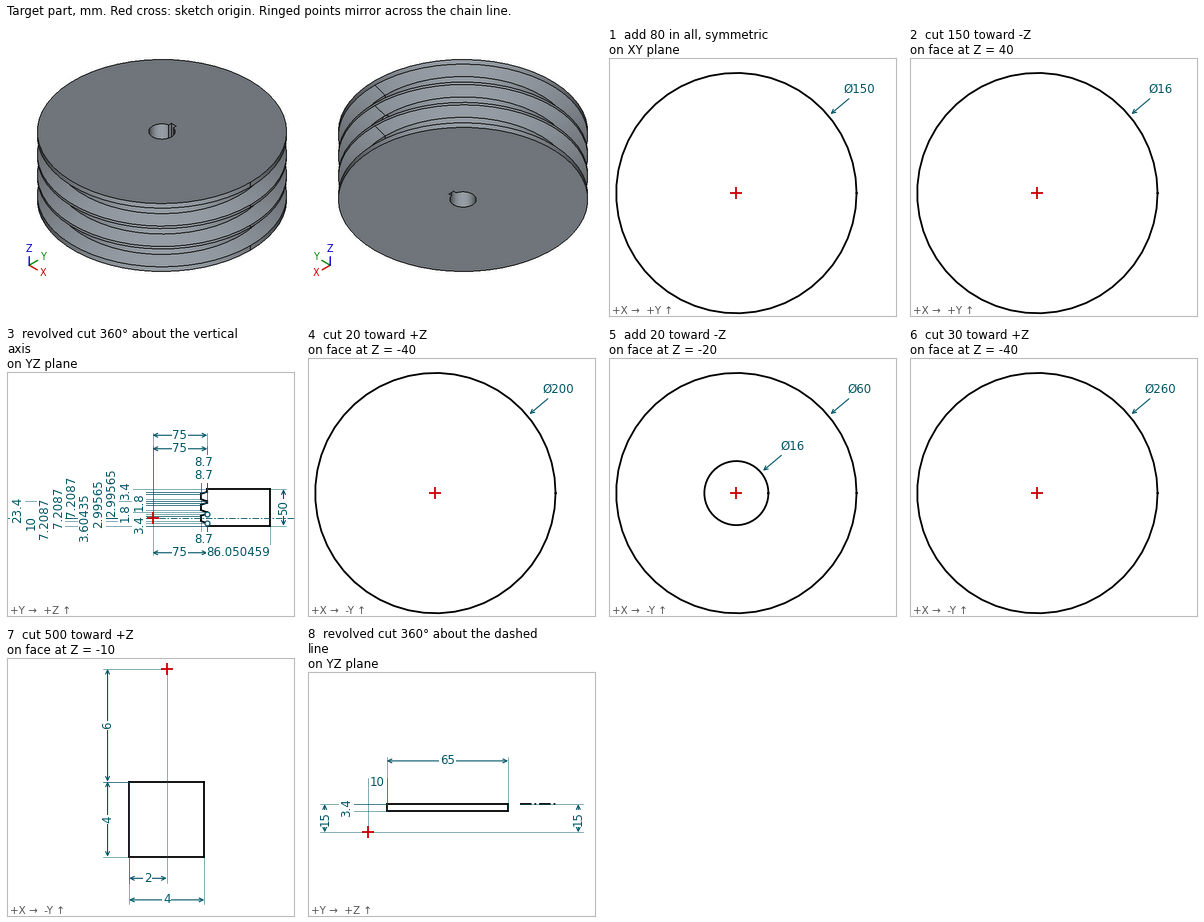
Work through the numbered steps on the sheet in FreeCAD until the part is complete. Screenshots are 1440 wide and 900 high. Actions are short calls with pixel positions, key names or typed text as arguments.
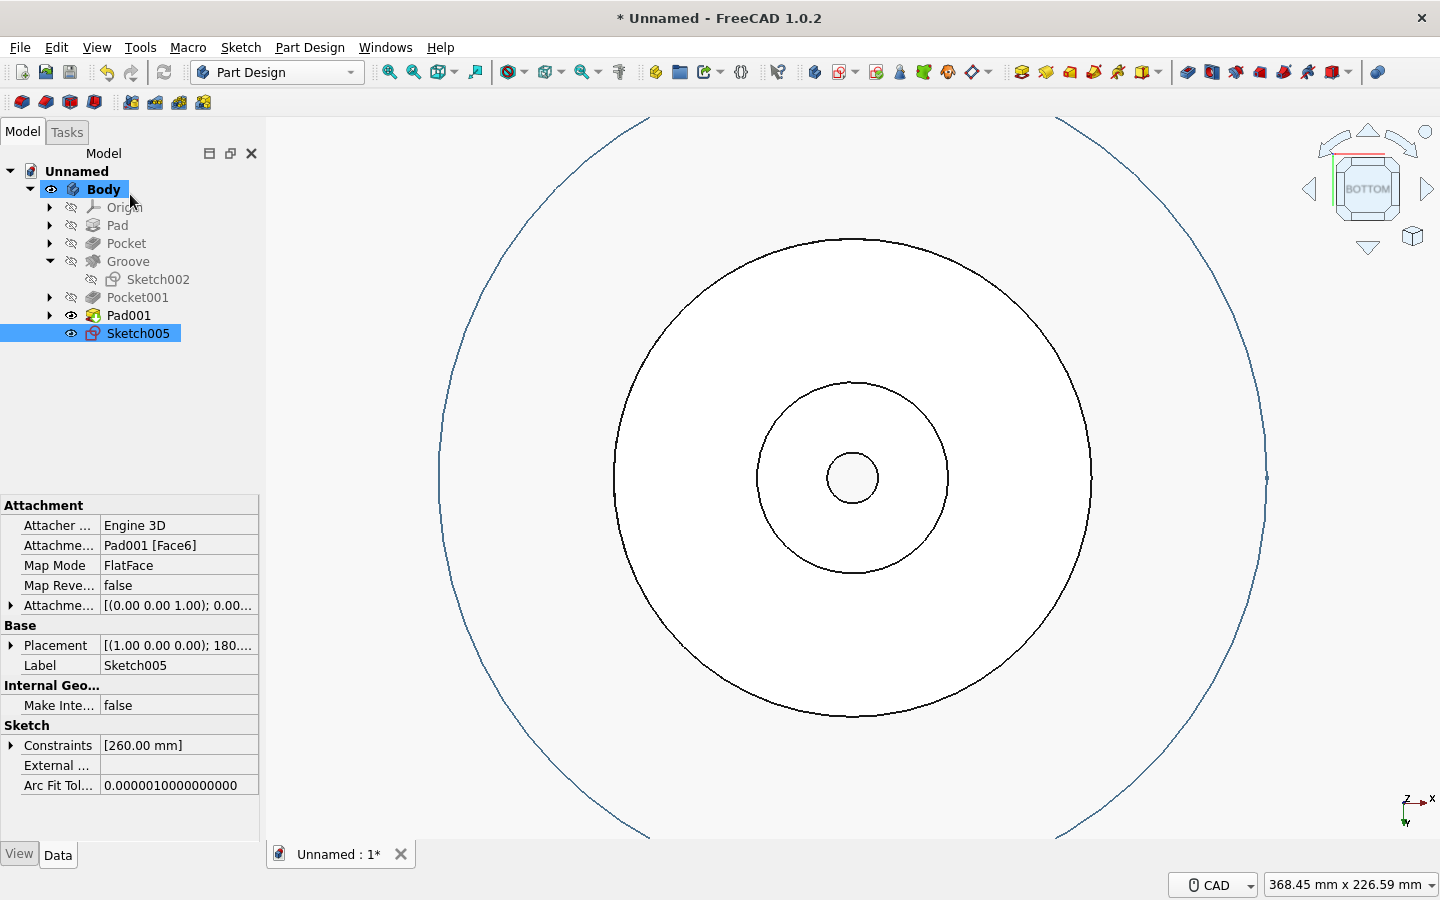
click(1188, 72)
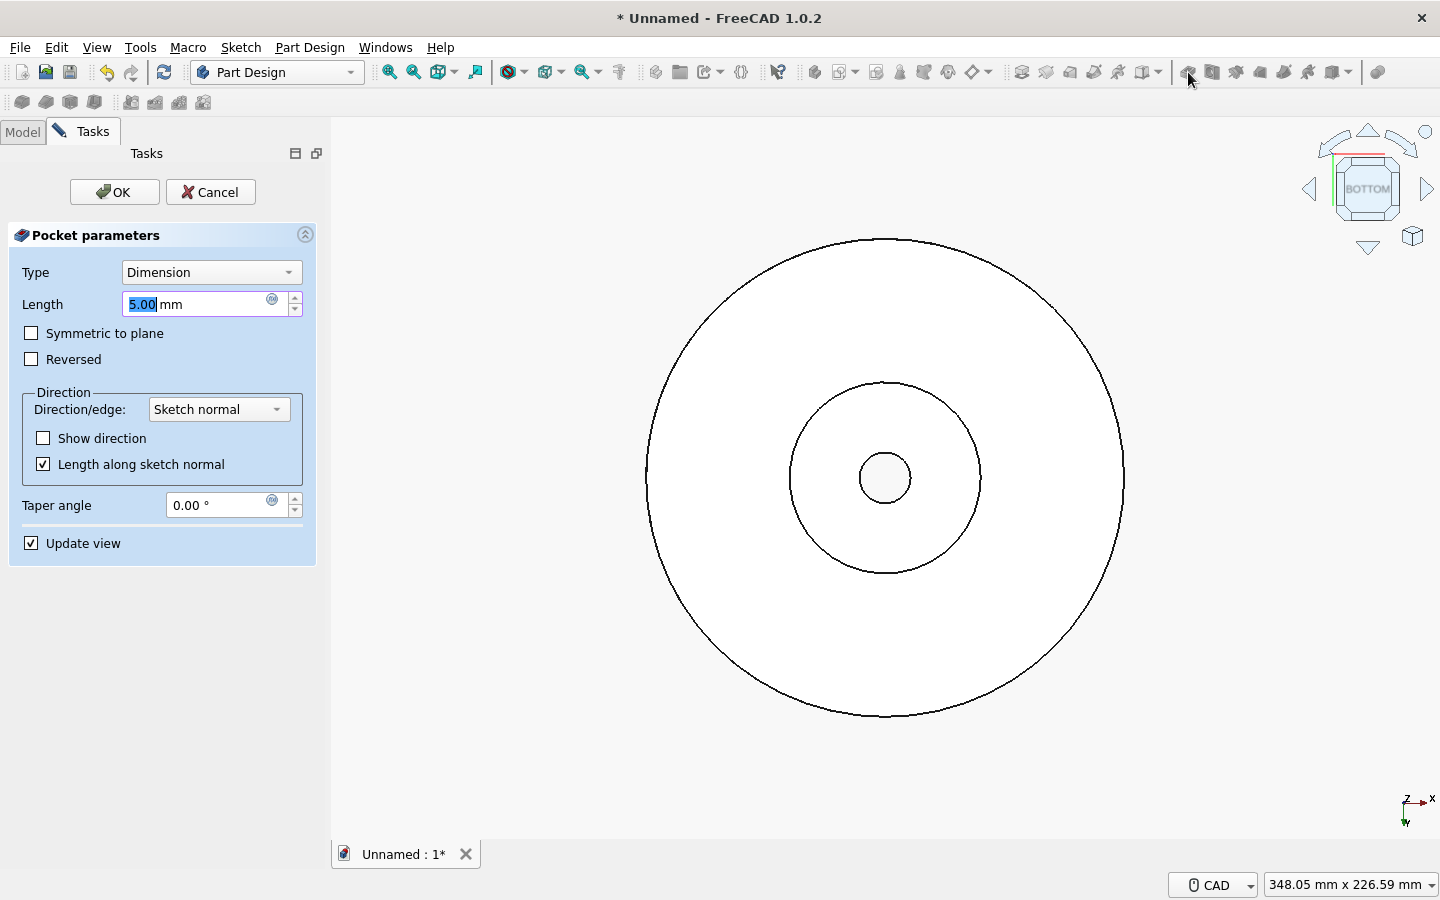
text(30)
key(Tab)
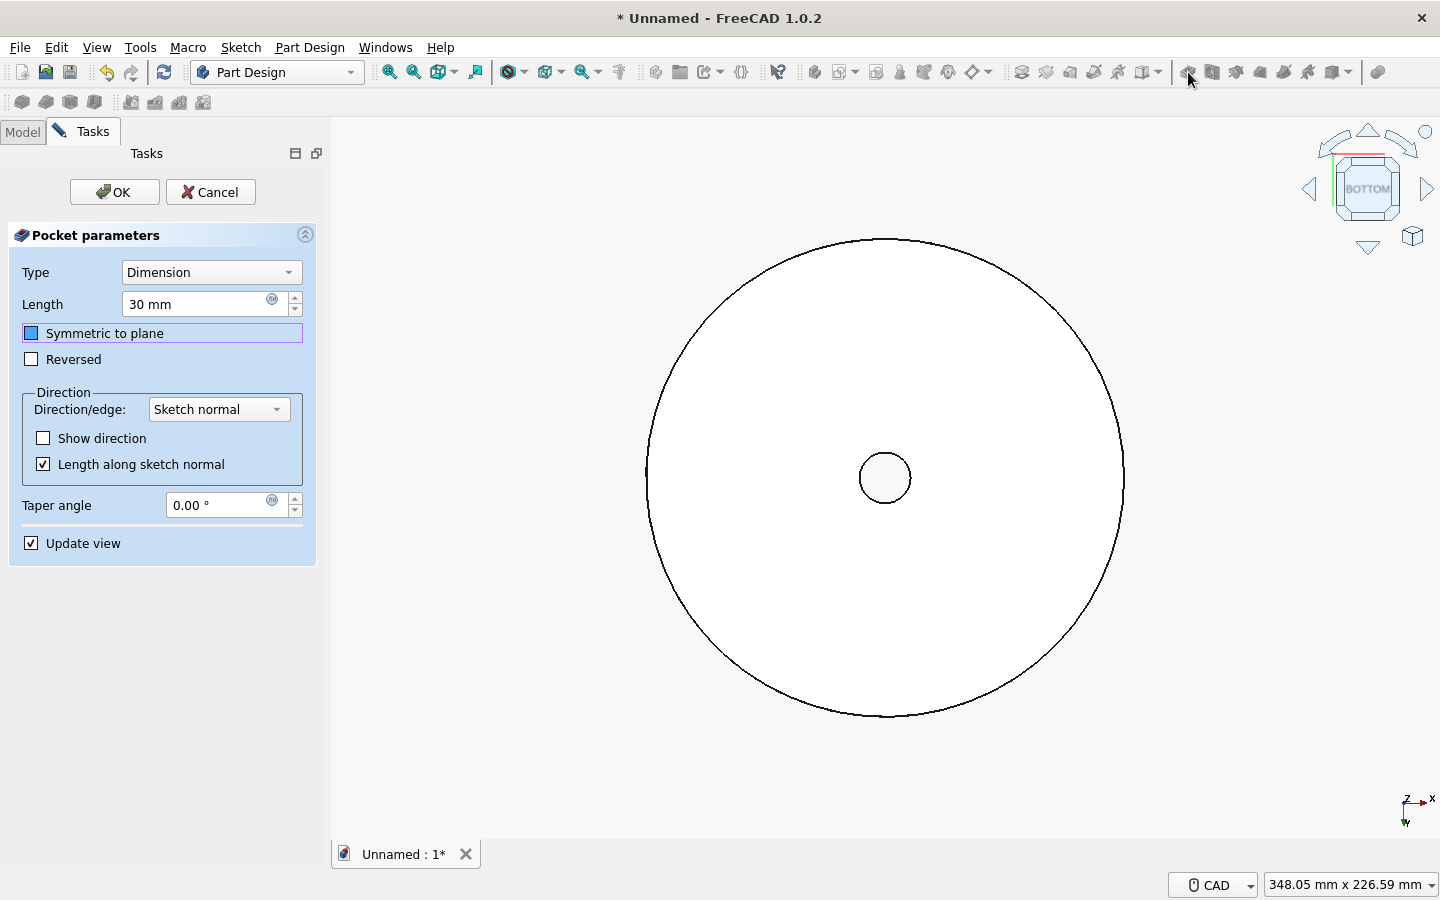
click(115, 192)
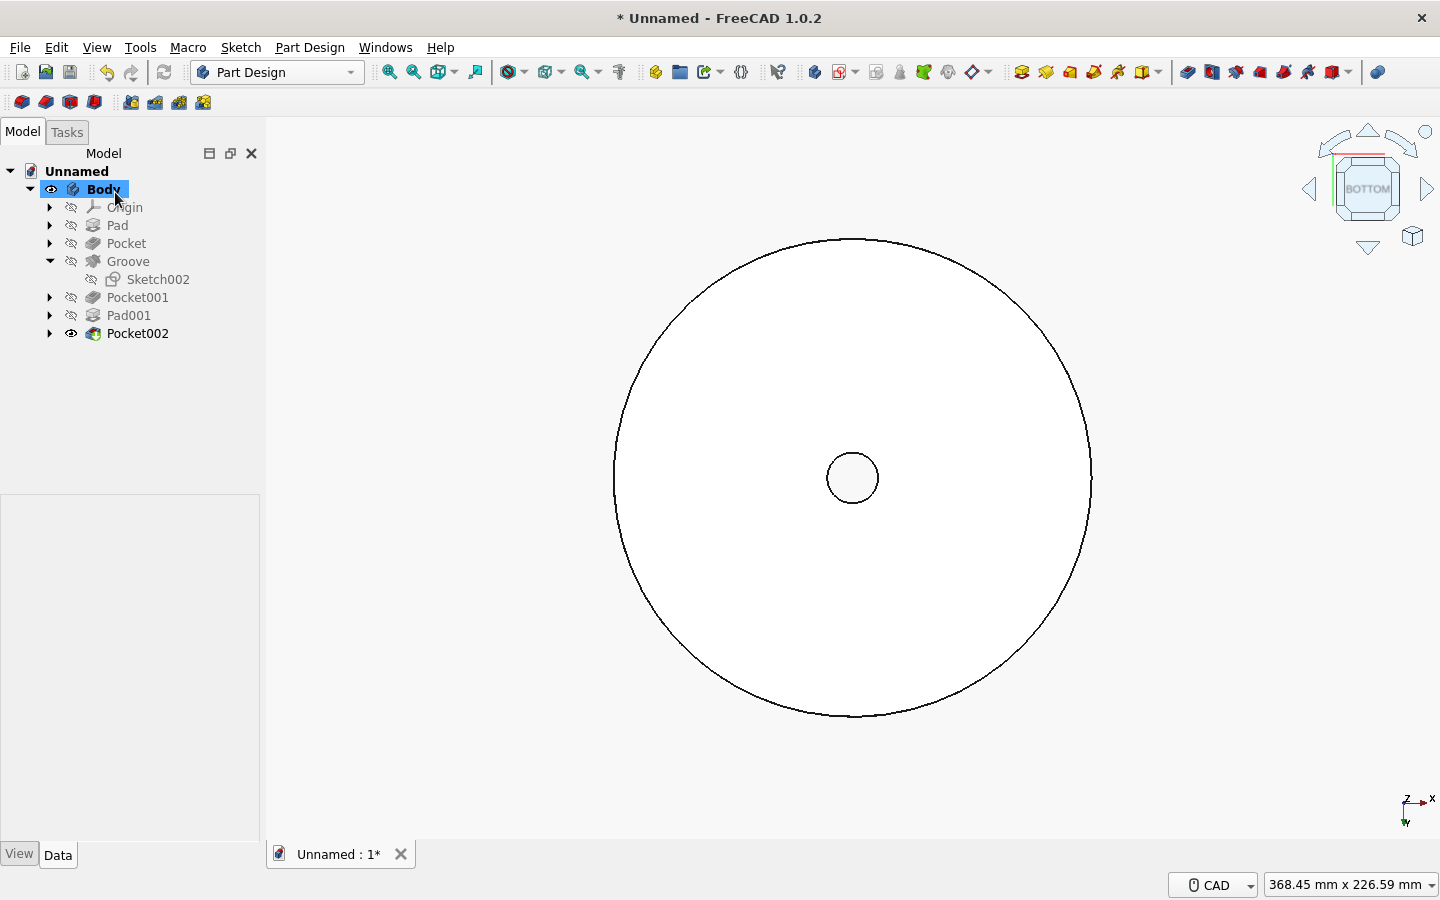
click(716, 477)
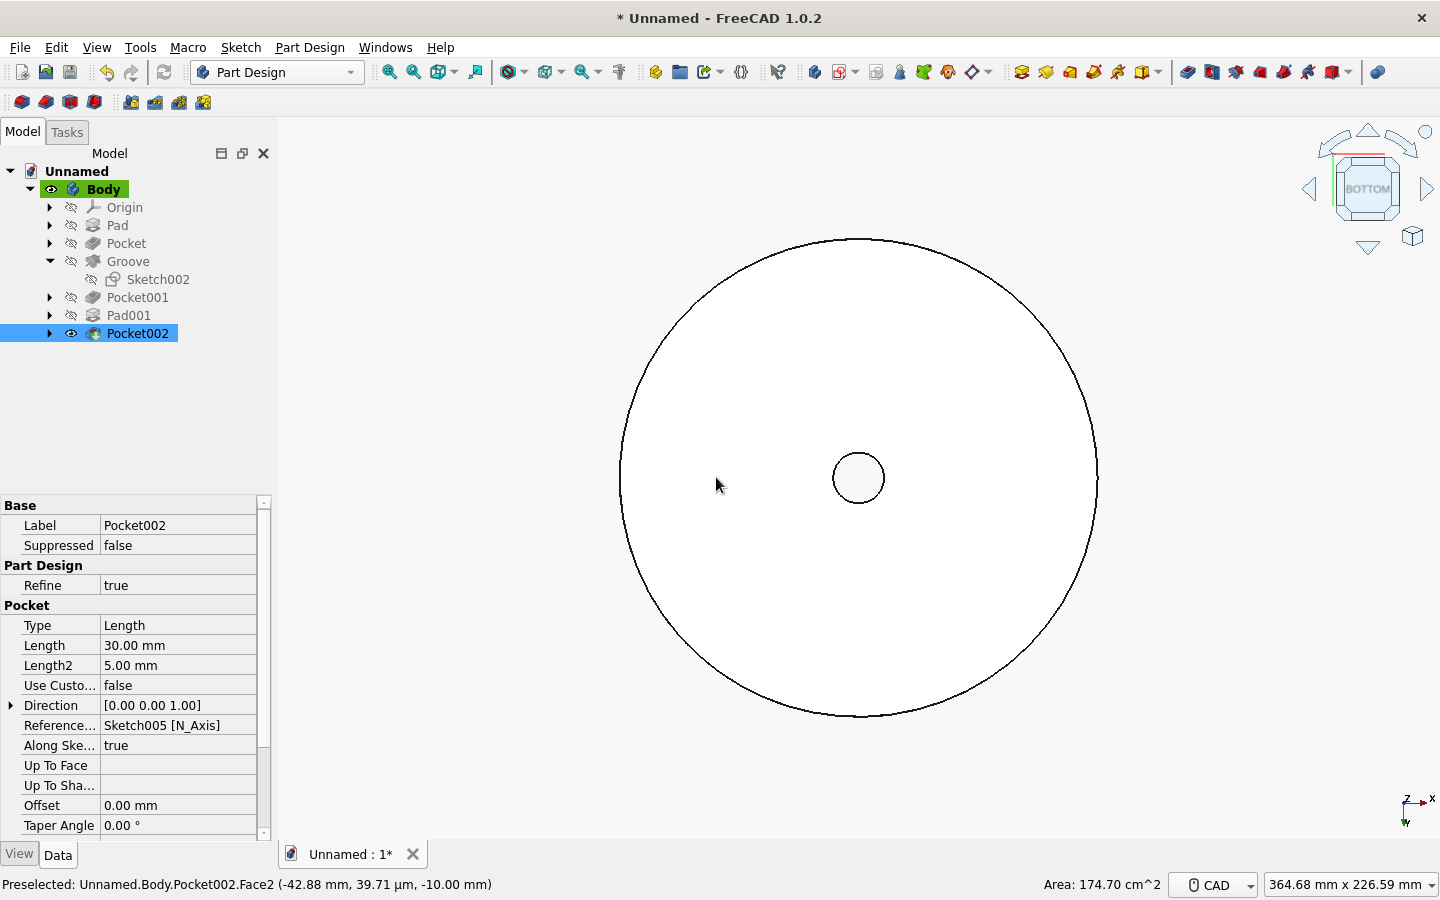
click(840, 72)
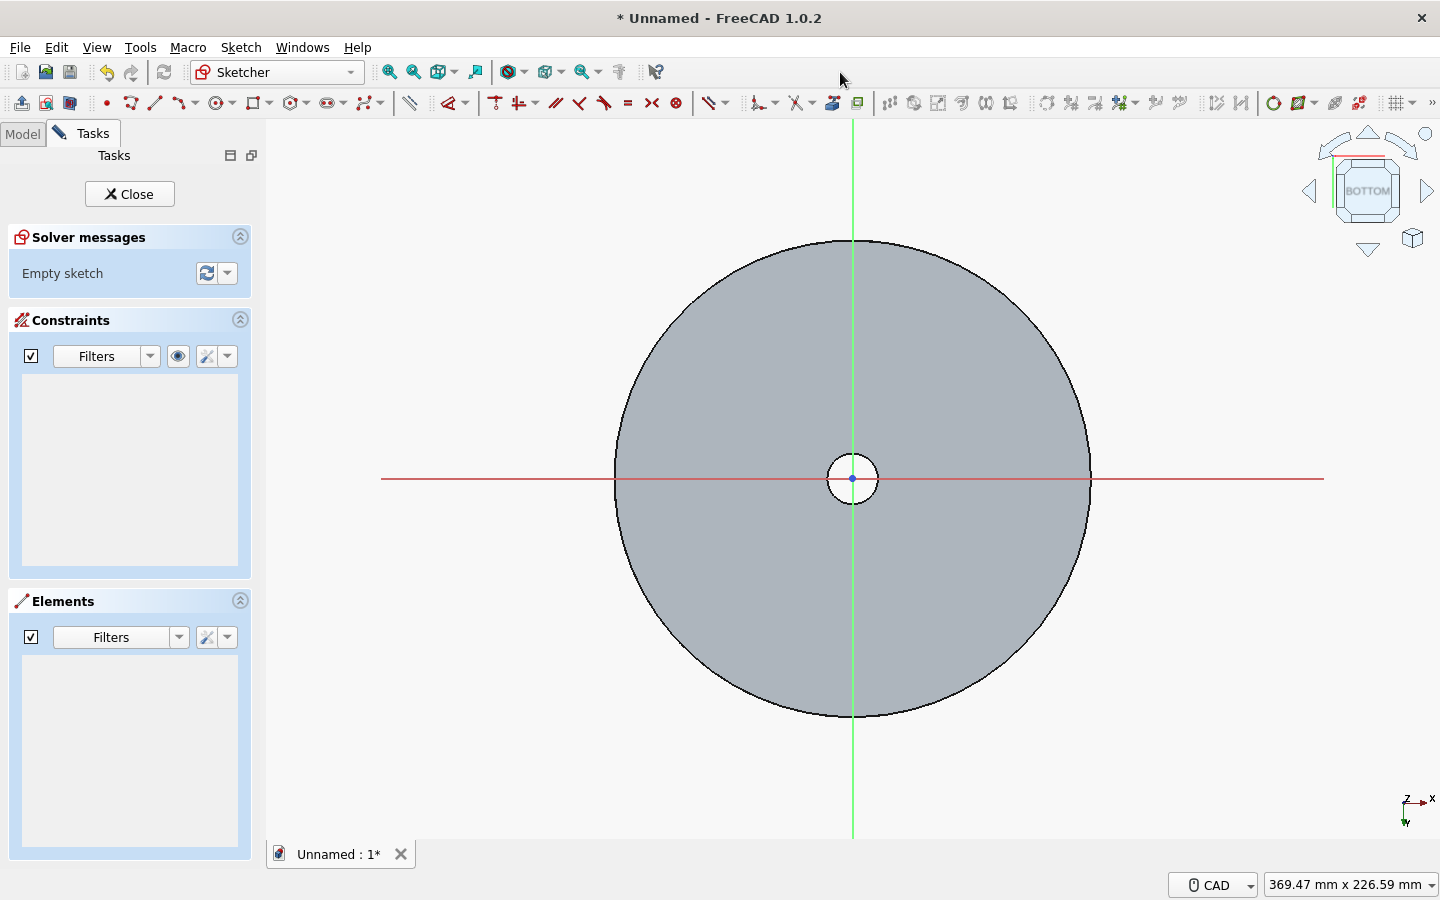
scroll(856, 506, up, 15)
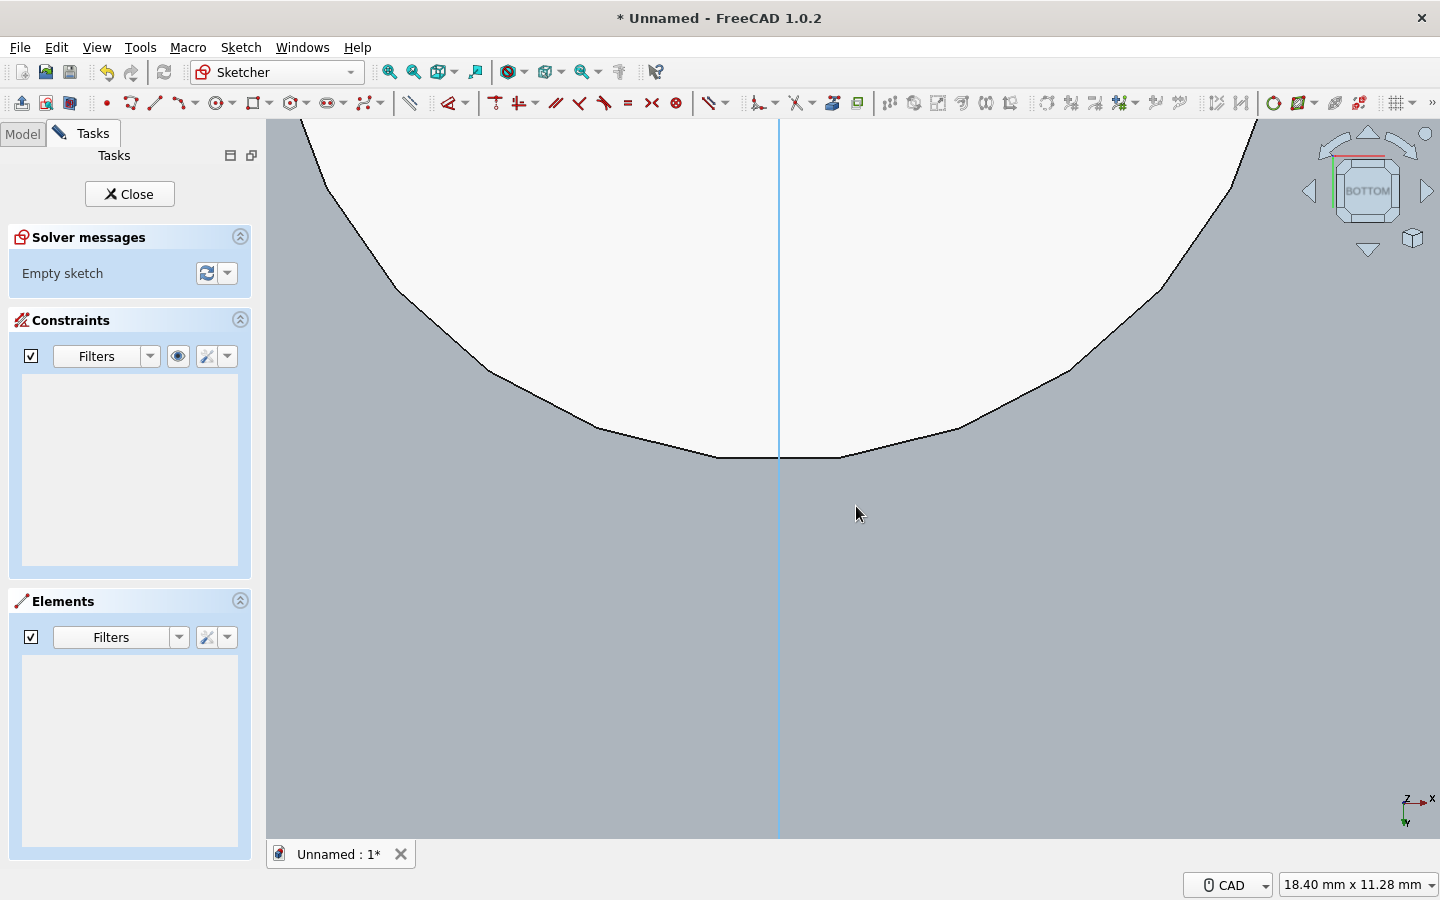
scroll(772, 440, up, 3)